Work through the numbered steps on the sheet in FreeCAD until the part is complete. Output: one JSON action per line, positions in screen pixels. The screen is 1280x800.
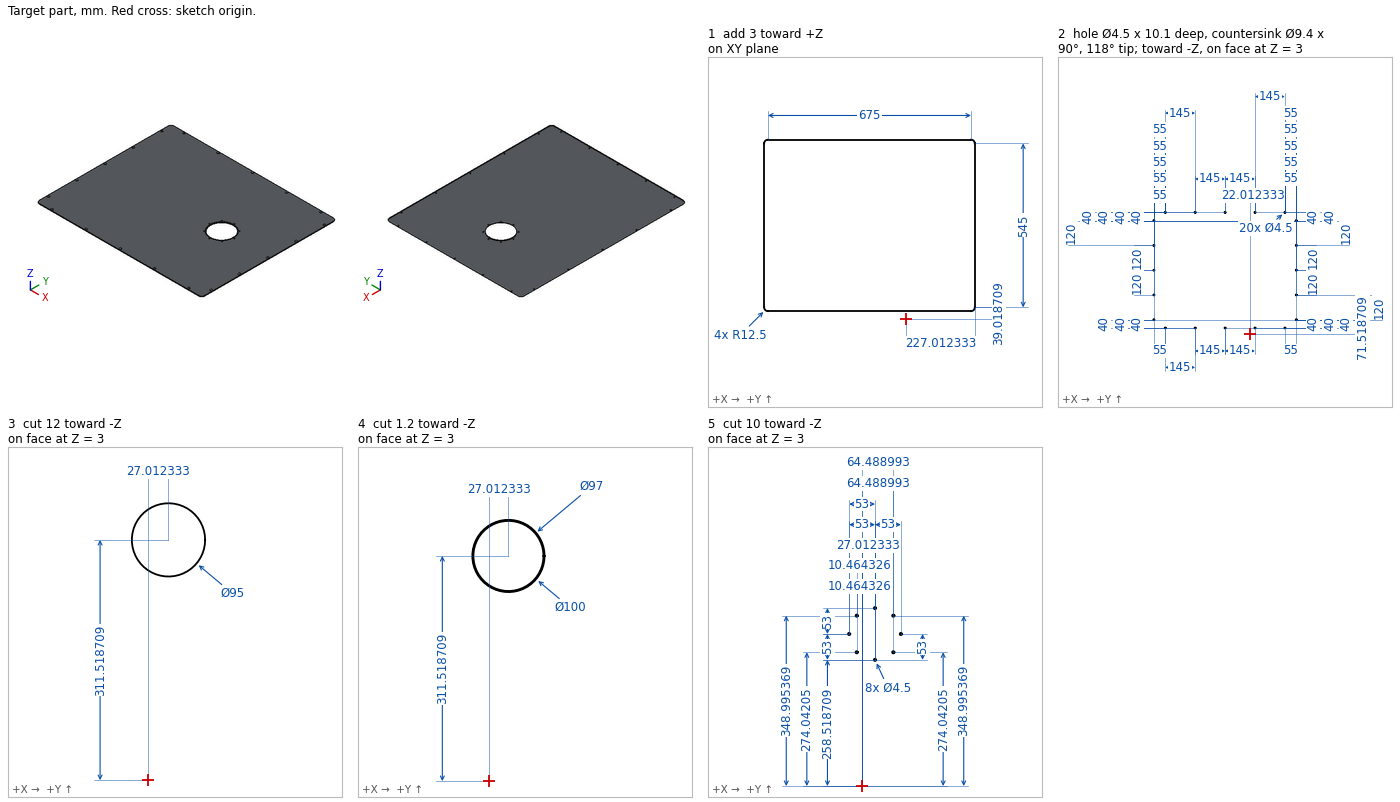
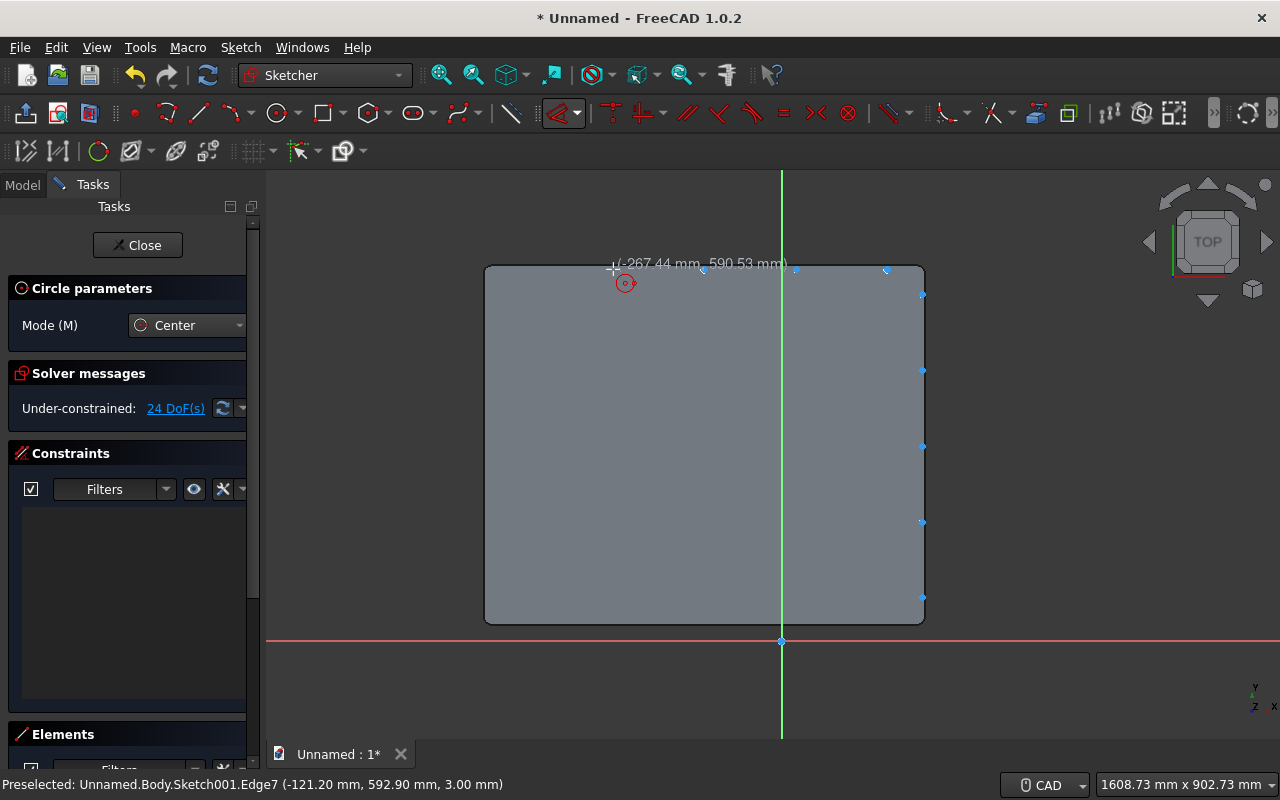
{"action": "left_click", "coordinate": [613, 269]}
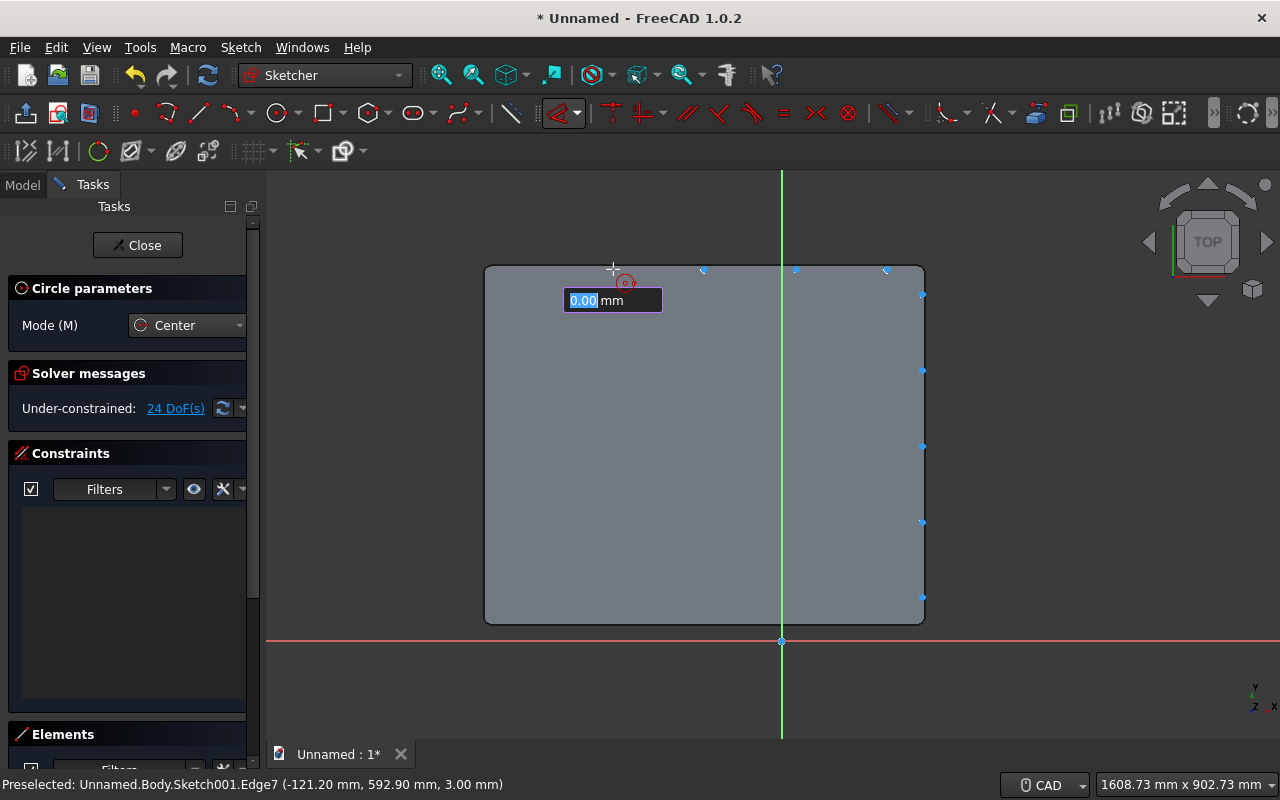
{"action": "scroll", "coordinate": [614, 268], "scroll_direction": "up", "scroll_amount": 13}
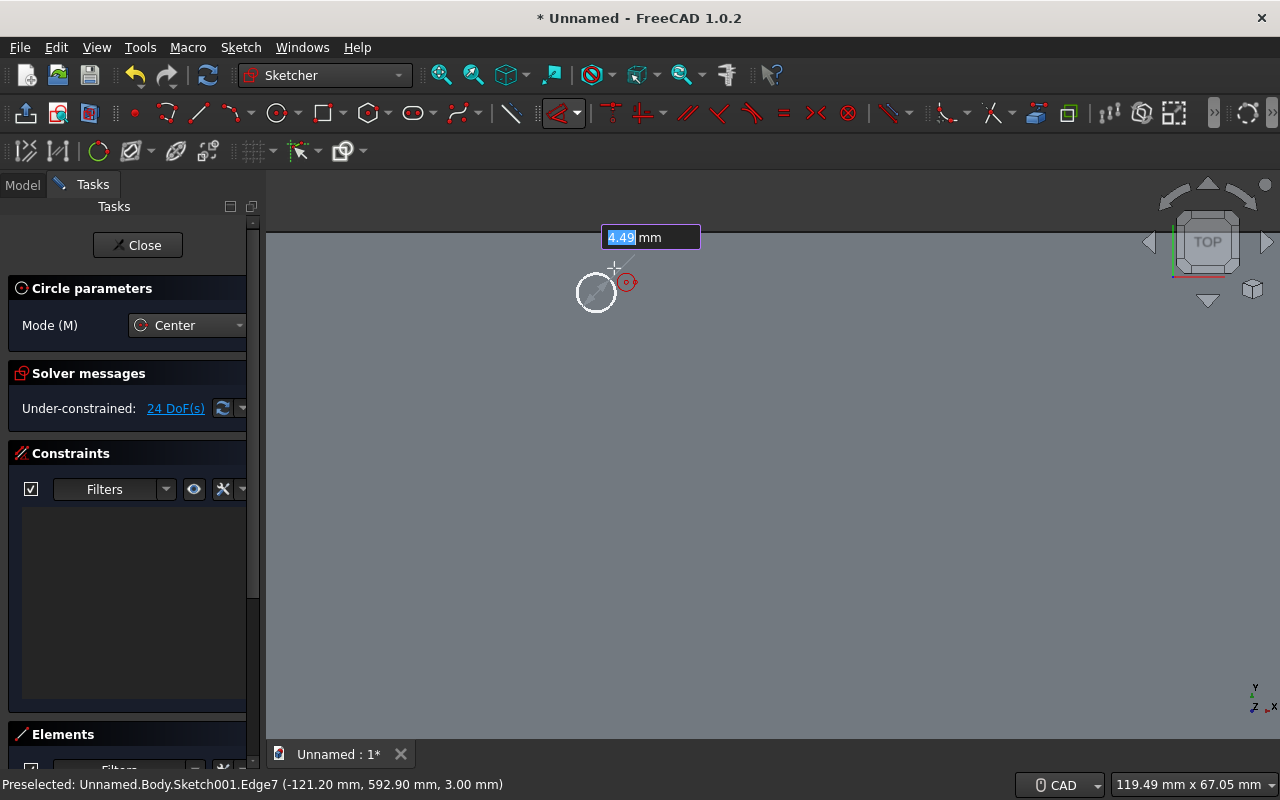
{"action": "left_click", "coordinate": [609, 260]}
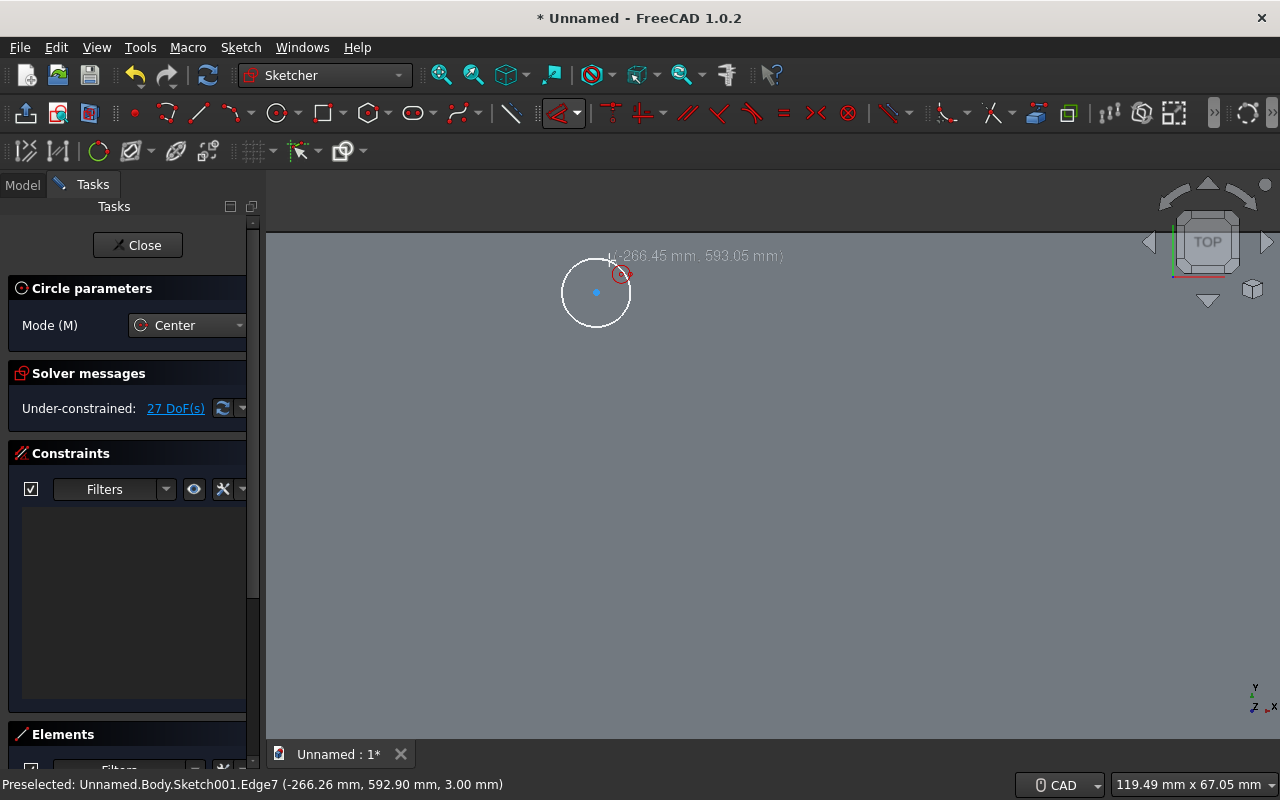
{"action": "scroll", "coordinate": [614, 268], "scroll_direction": "down", "scroll_amount": 13}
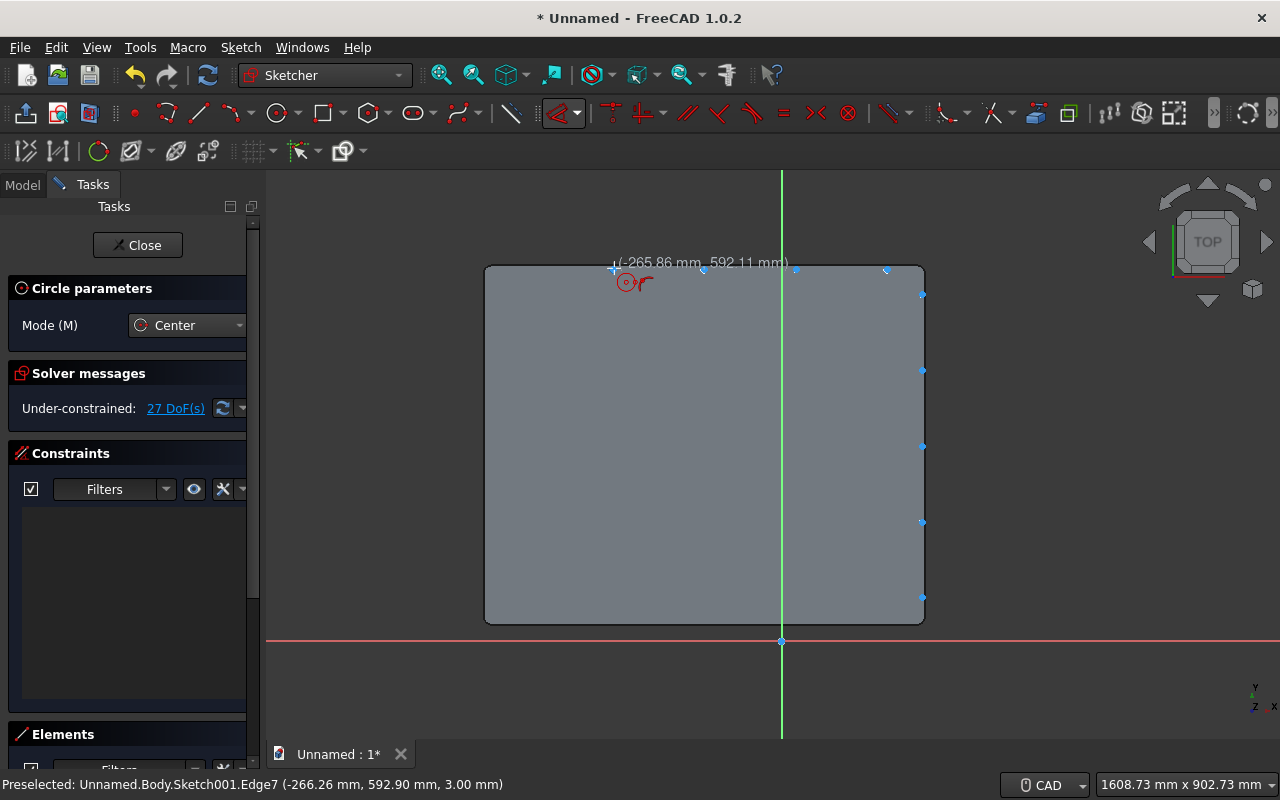
{"action": "scroll", "coordinate": [522, 269], "scroll_direction": "up", "scroll_amount": 14}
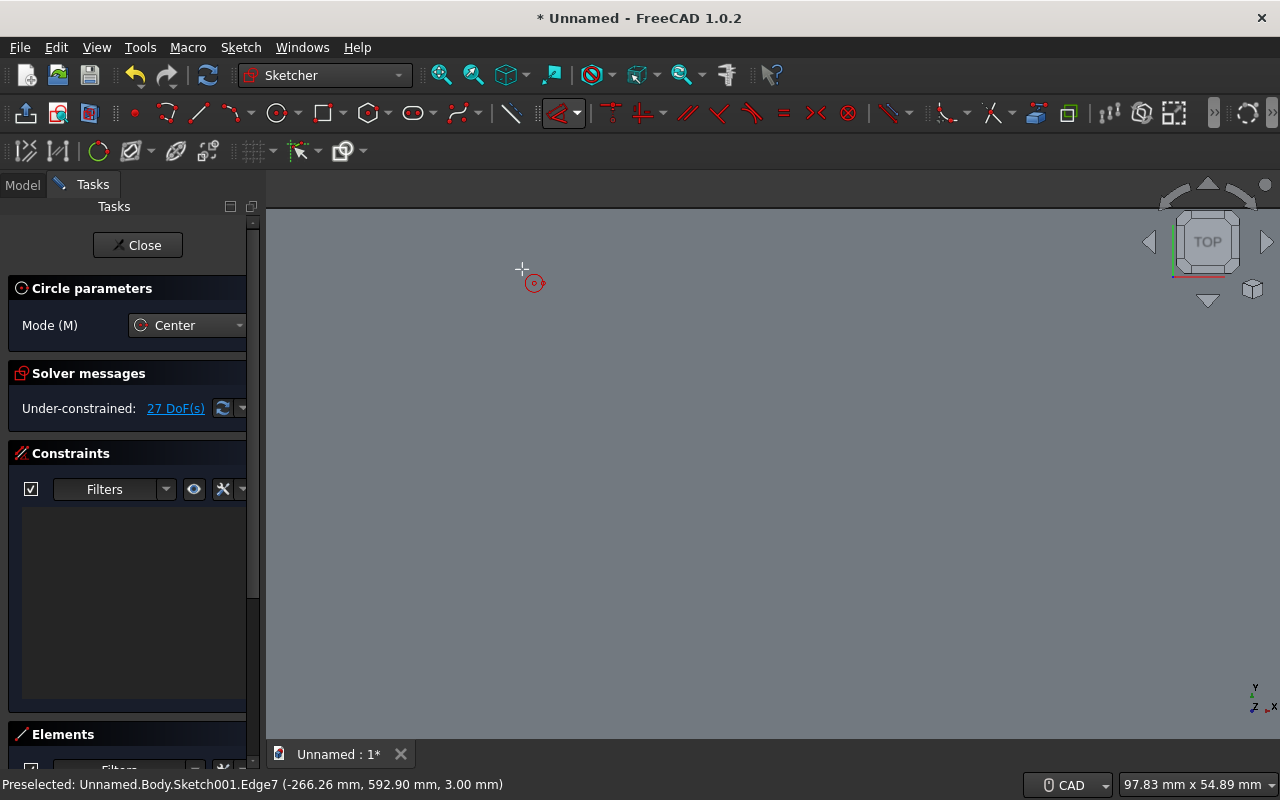
{"action": "scroll", "coordinate": [522, 269], "scroll_direction": "down", "scroll_amount": 14}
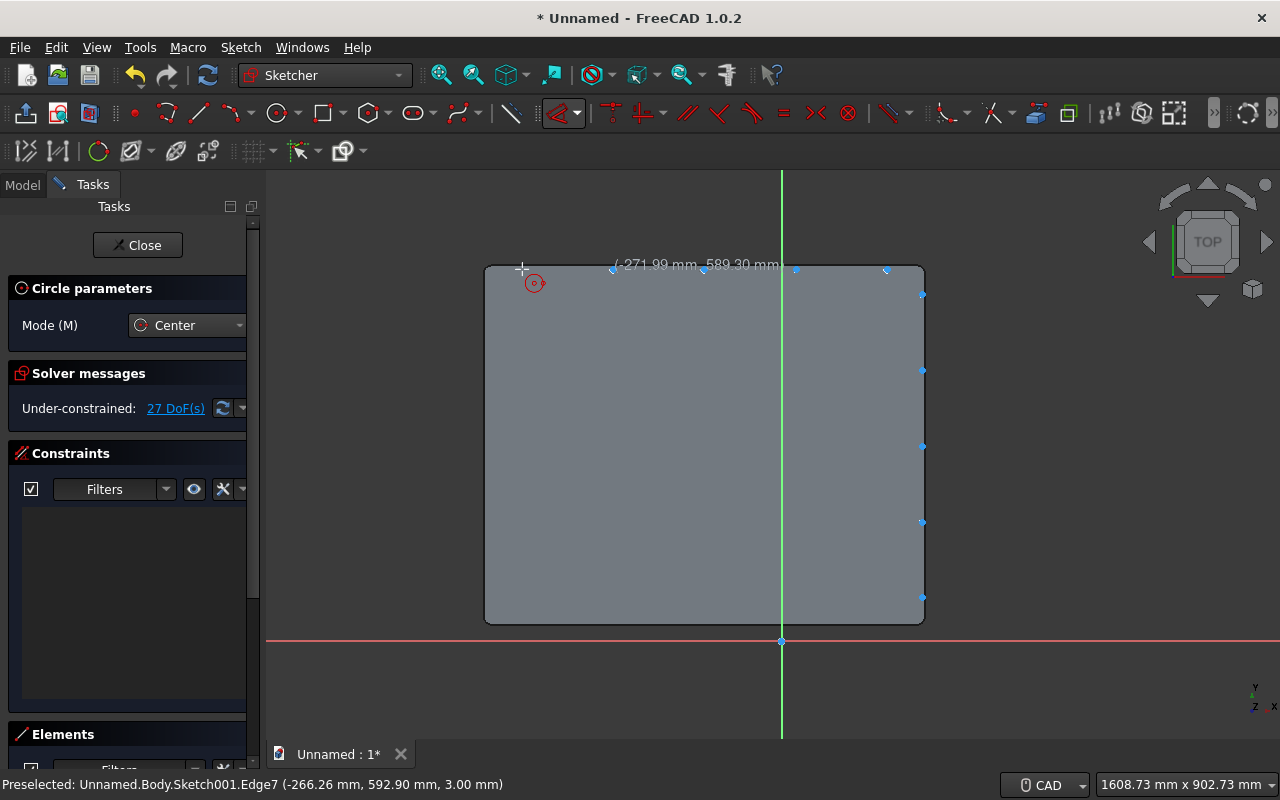
{"action": "left_click", "coordinate": [522, 269]}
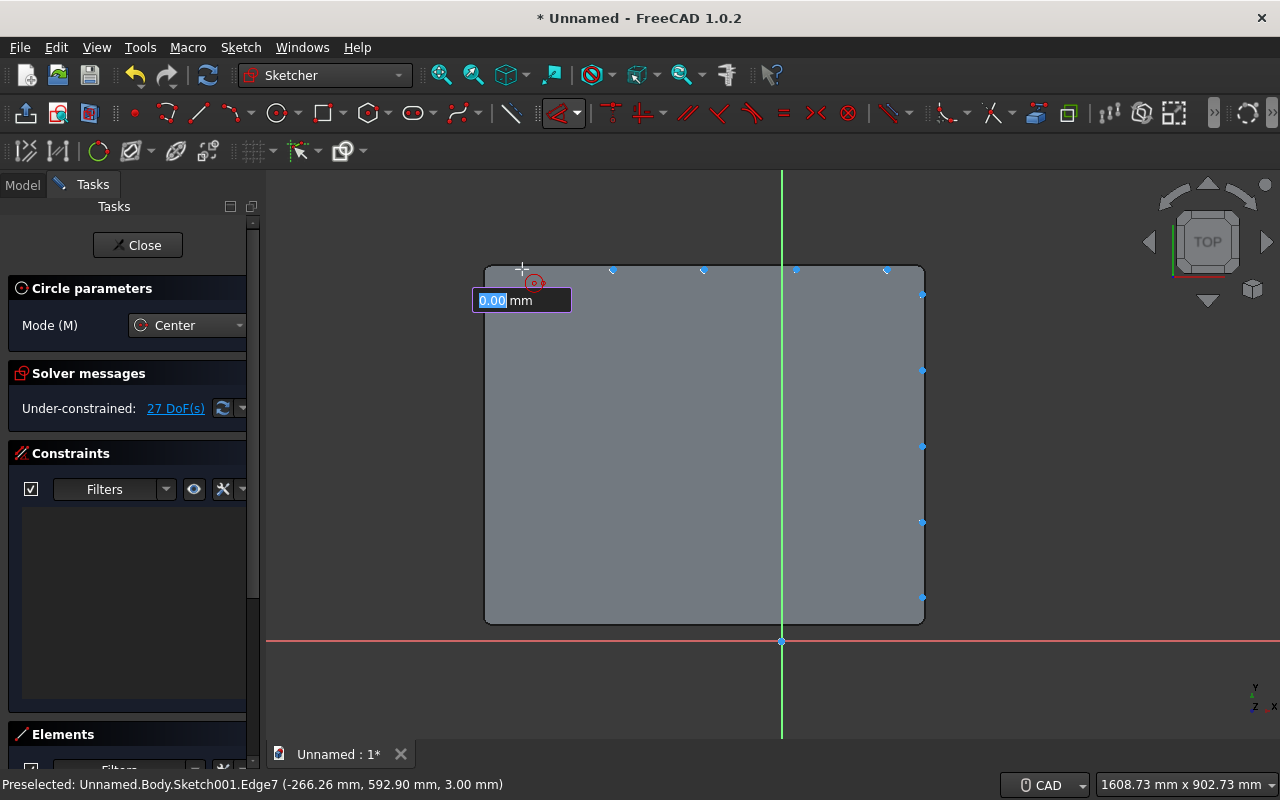
{"action": "scroll", "coordinate": [523, 268], "scroll_direction": "up", "scroll_amount": 13}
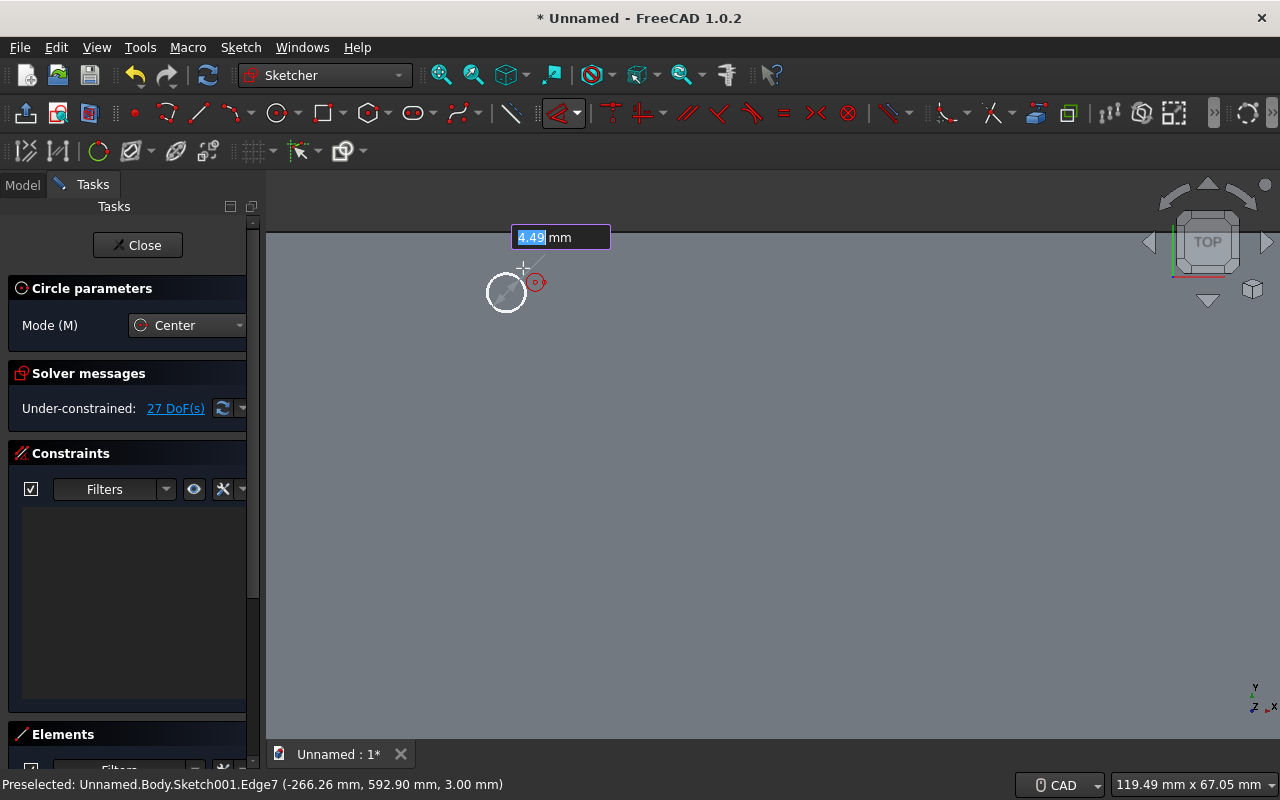
{"action": "left_click", "coordinate": [514, 260]}